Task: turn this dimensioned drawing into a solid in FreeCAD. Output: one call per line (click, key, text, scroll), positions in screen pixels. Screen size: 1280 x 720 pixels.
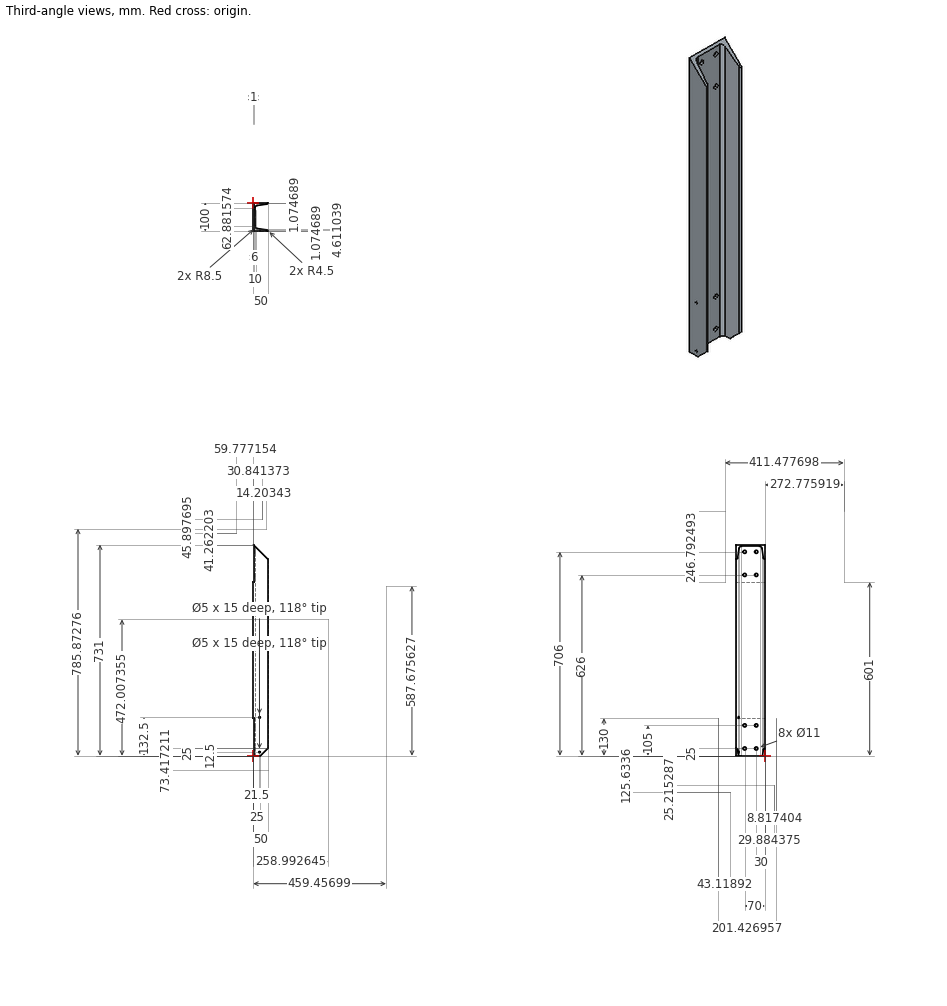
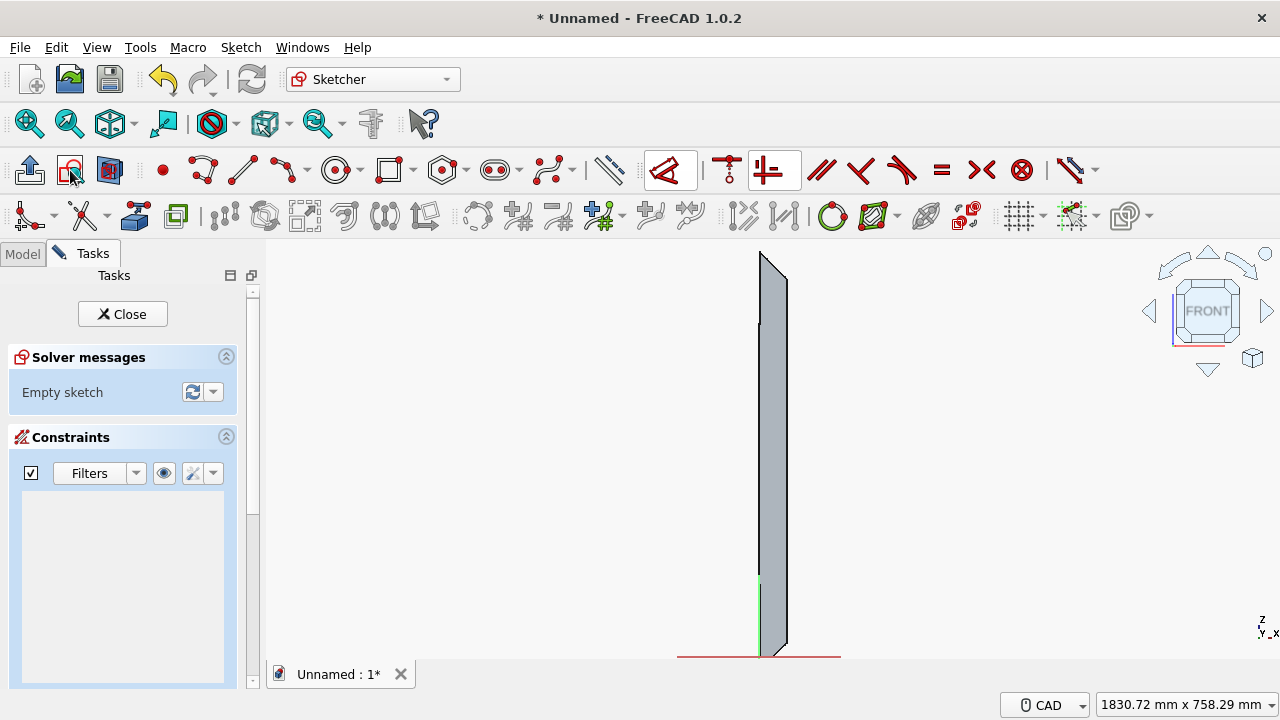
scroll(704, 449, down, 5)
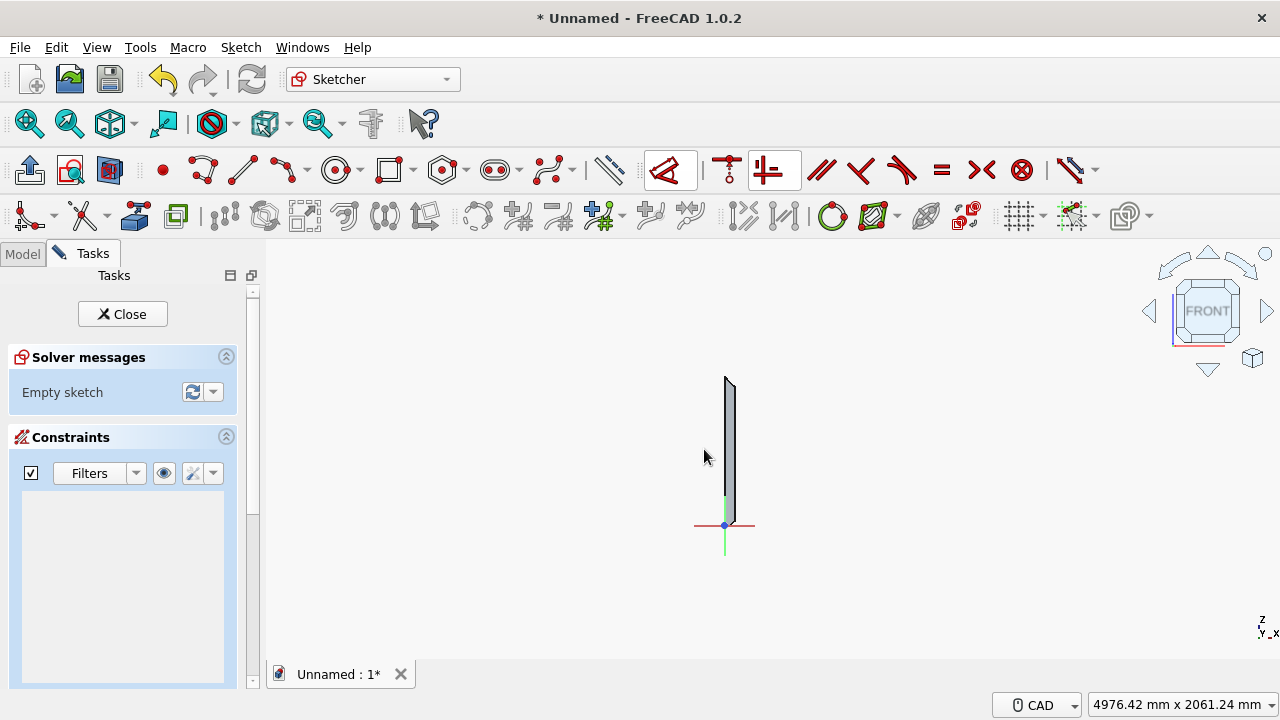
scroll(730, 527, up, 15)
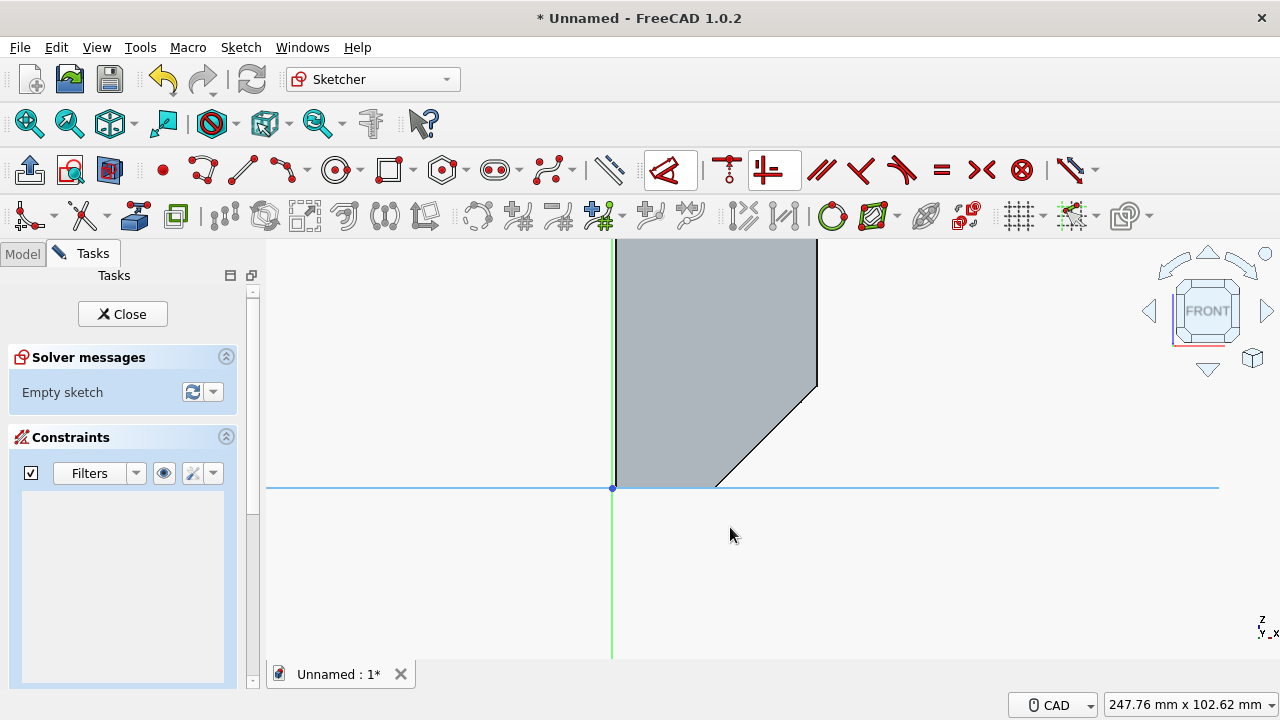
scroll(700, 436, up, 13)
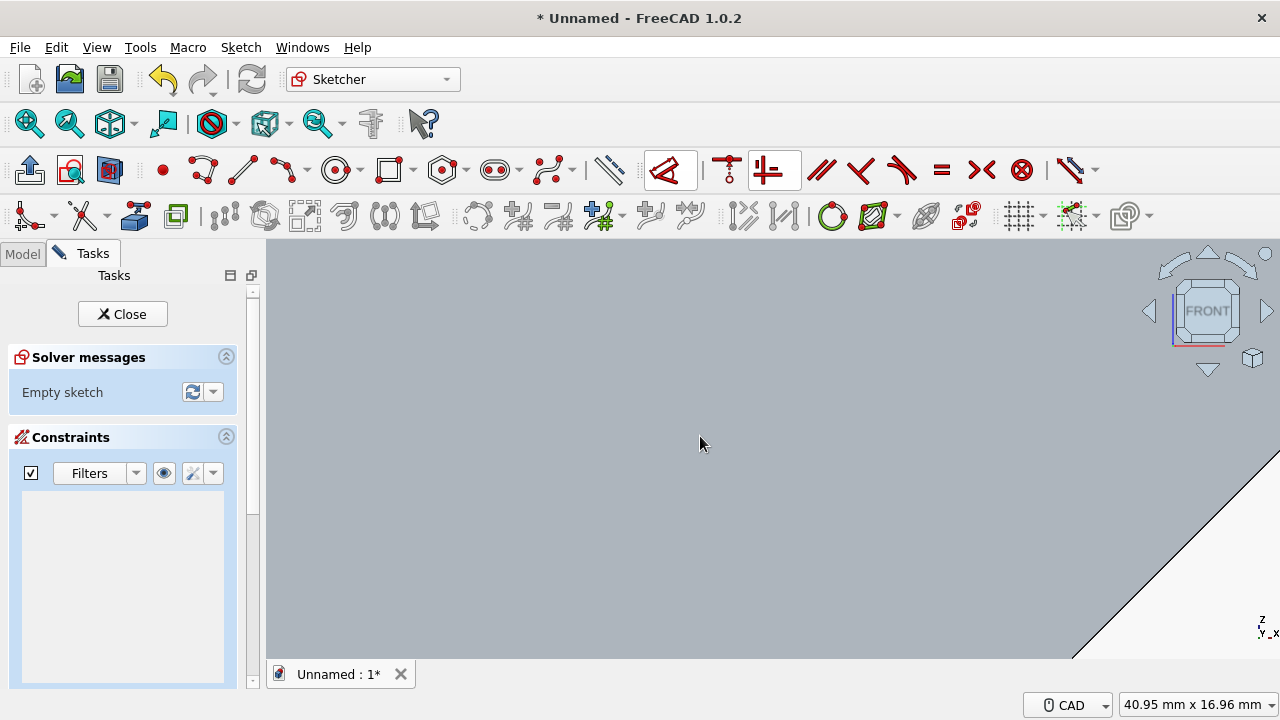
click(336, 170)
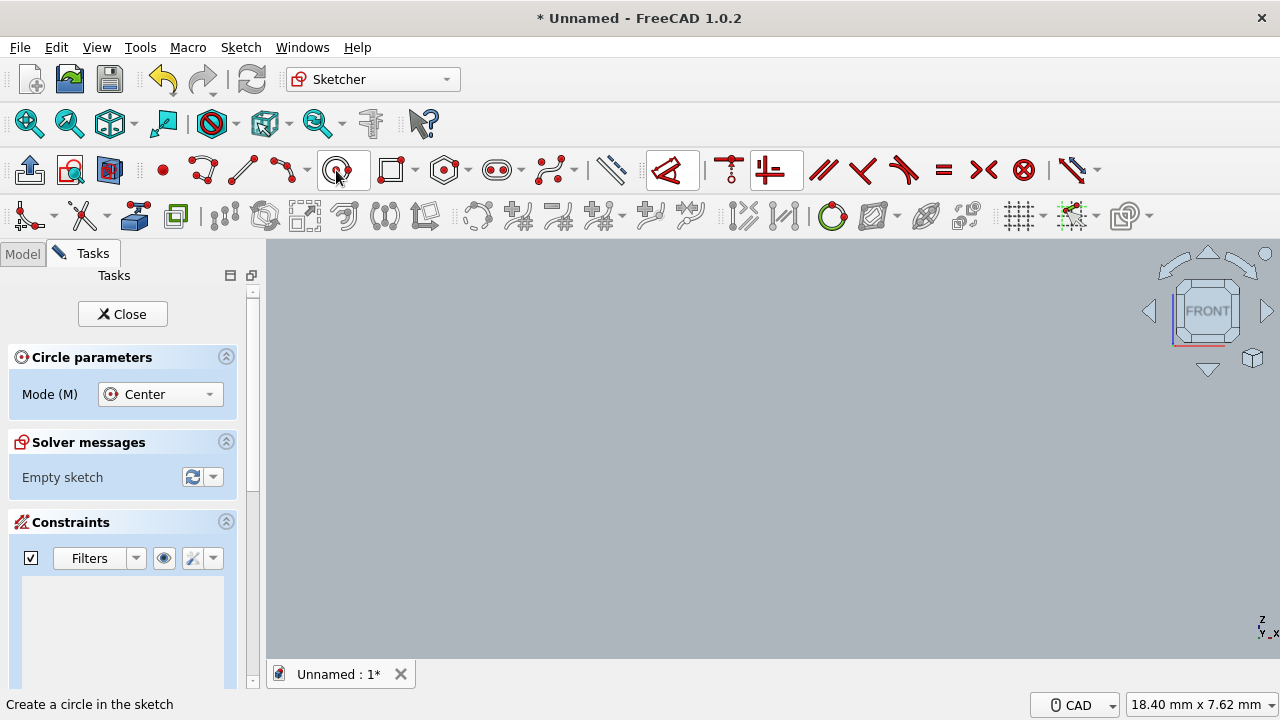
click(695, 446)
move(793, 348)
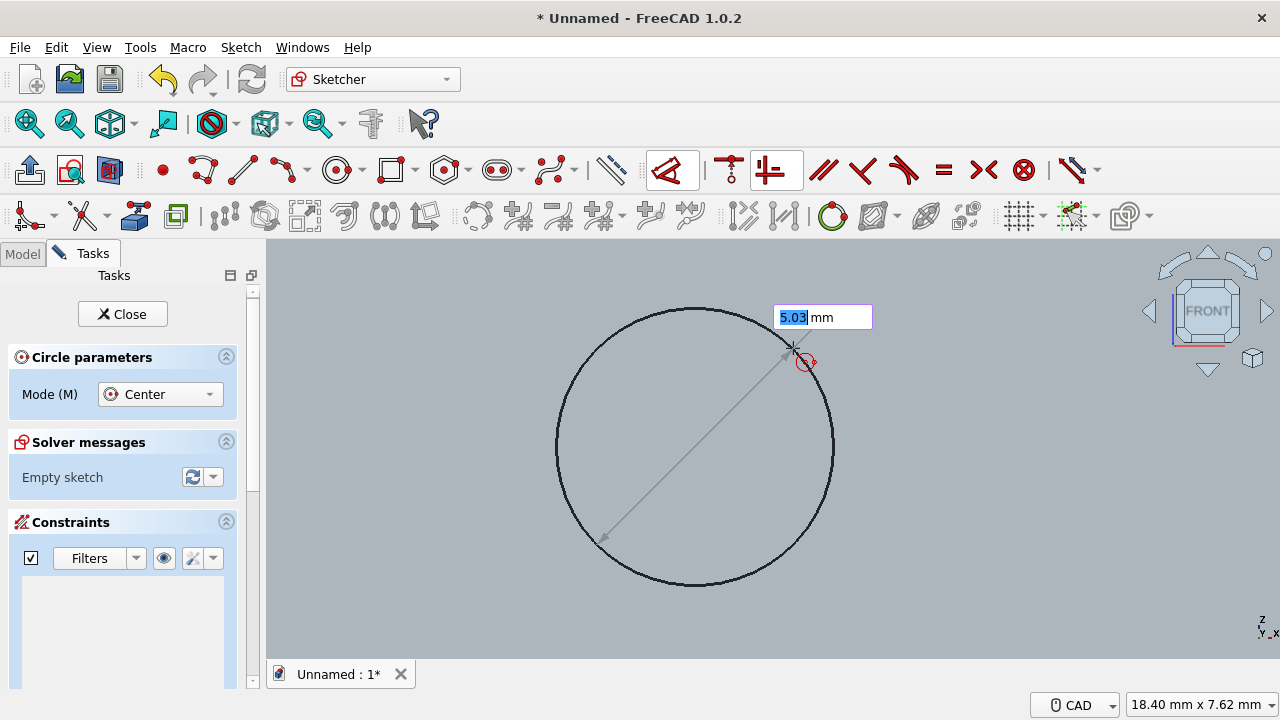
text(5)
key(Return)
key(Escape)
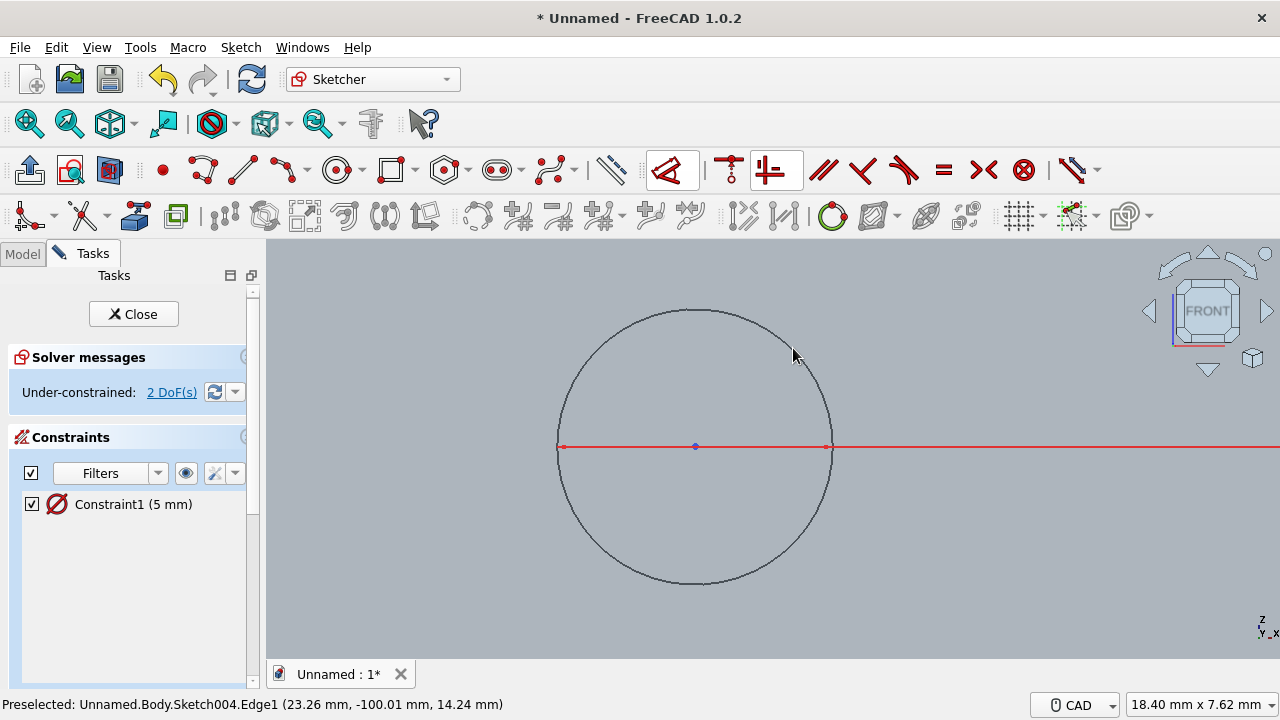
click(695, 447)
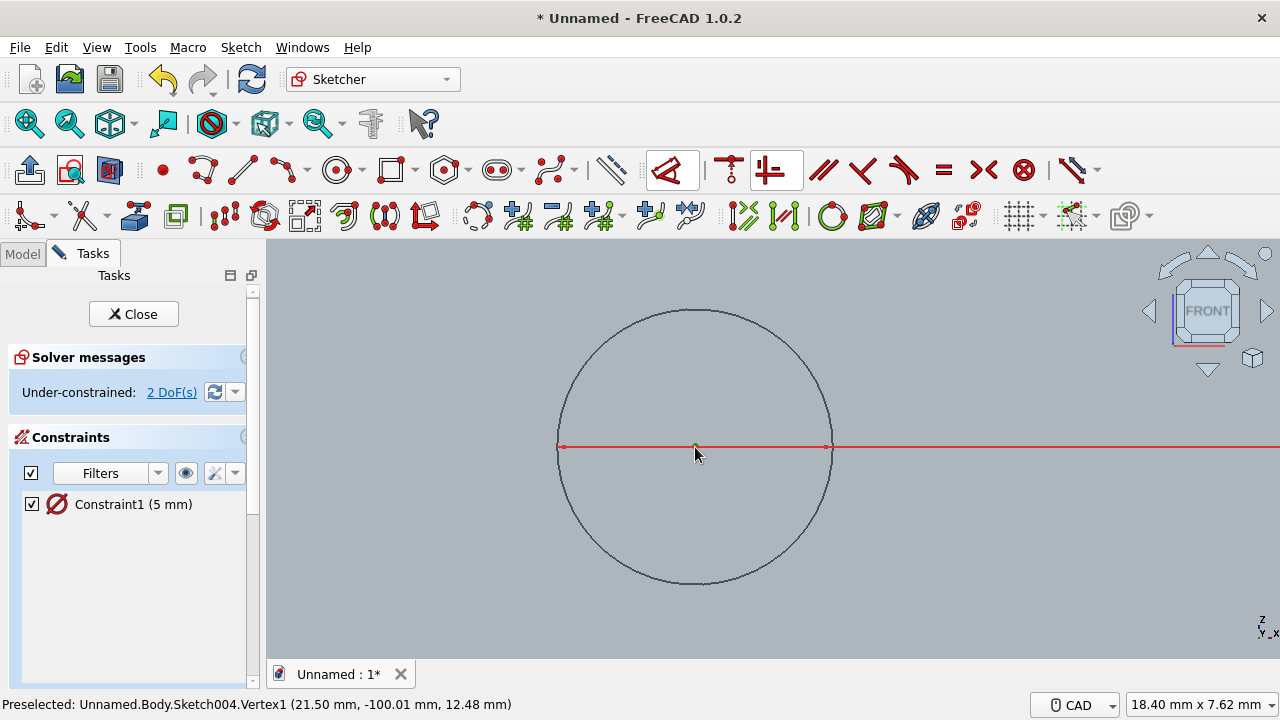
key(l)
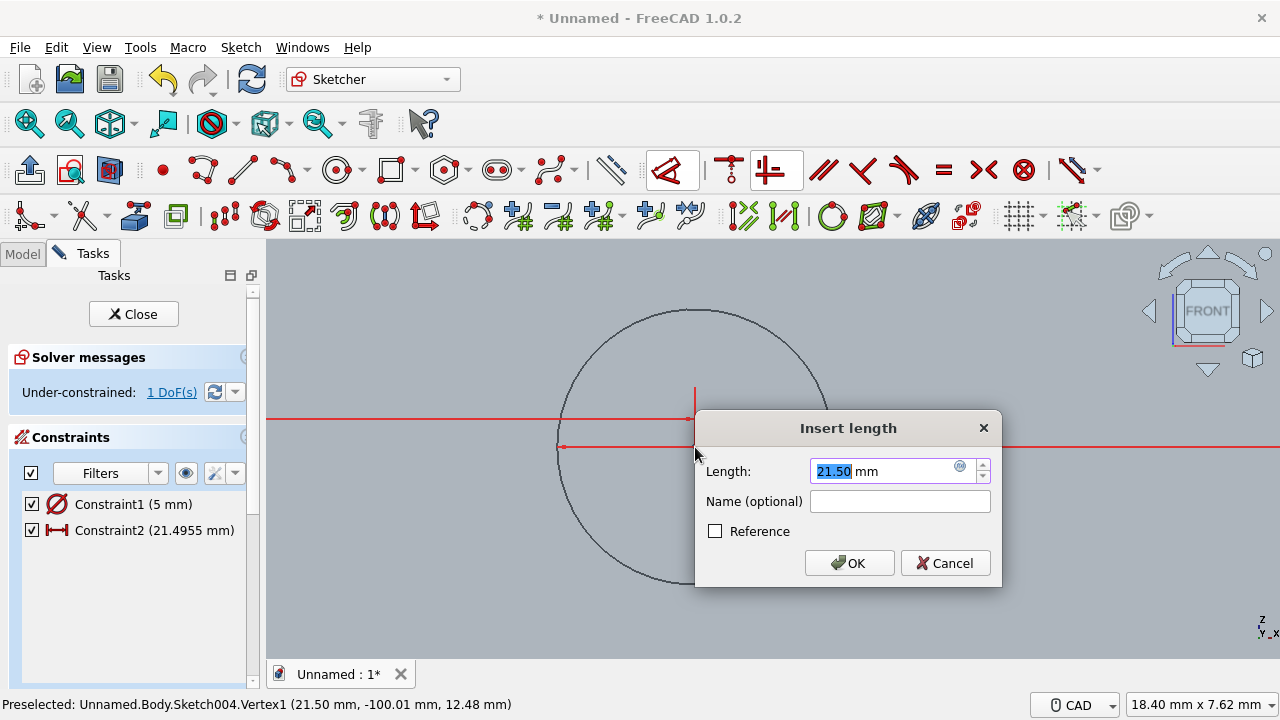
text(21.5)
key(Return)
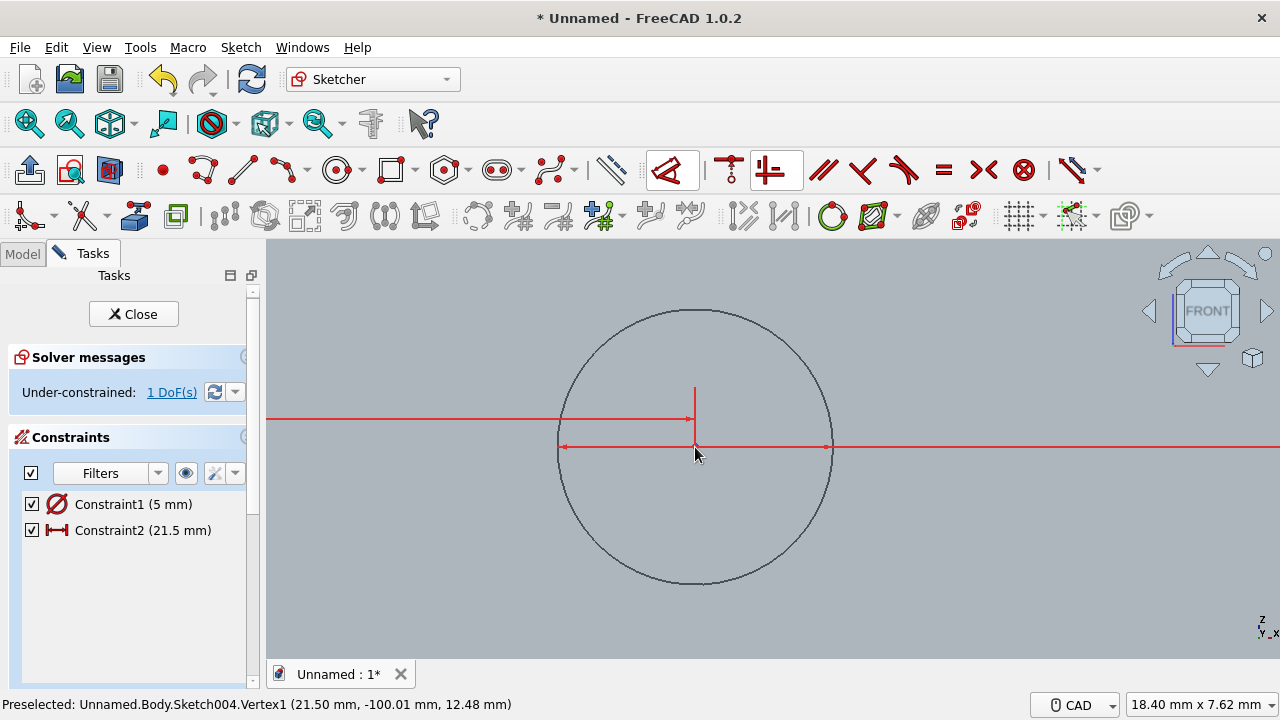
click(695, 447)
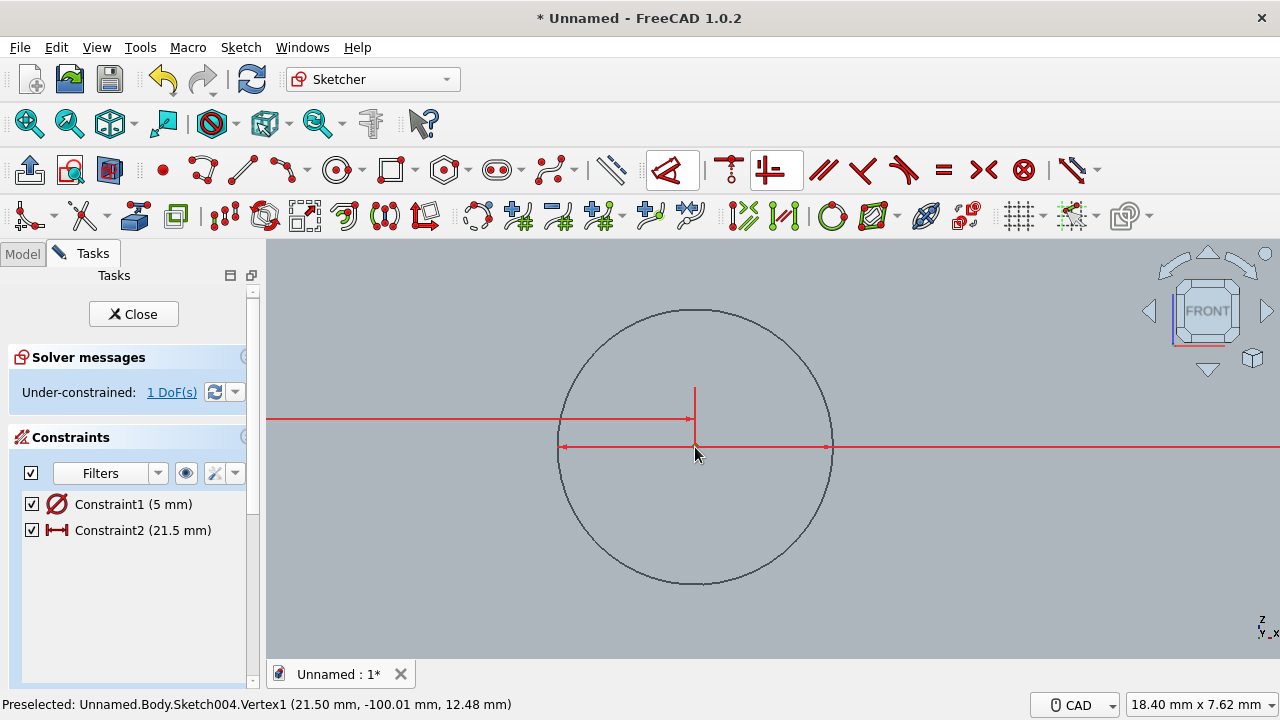
key(i)